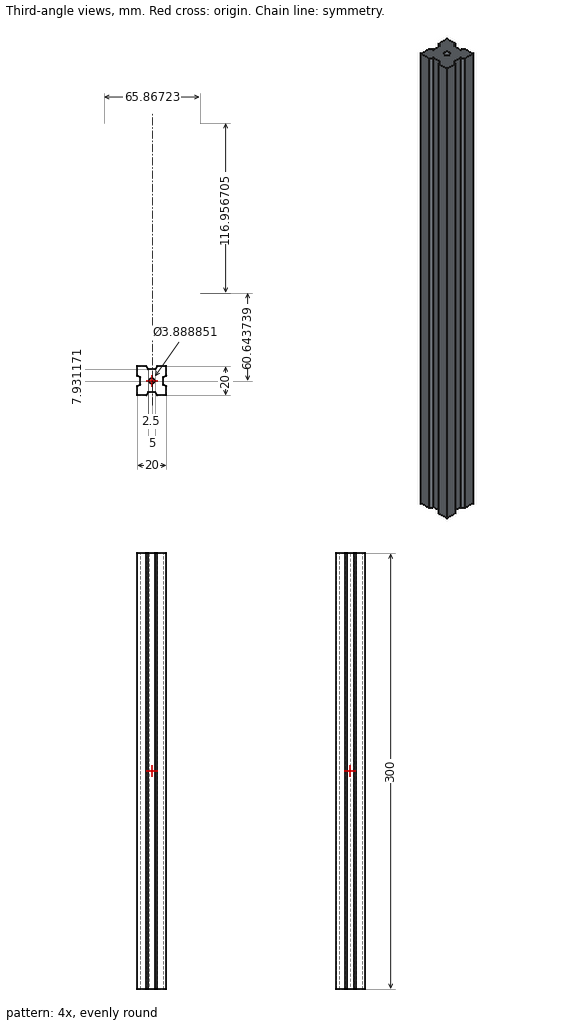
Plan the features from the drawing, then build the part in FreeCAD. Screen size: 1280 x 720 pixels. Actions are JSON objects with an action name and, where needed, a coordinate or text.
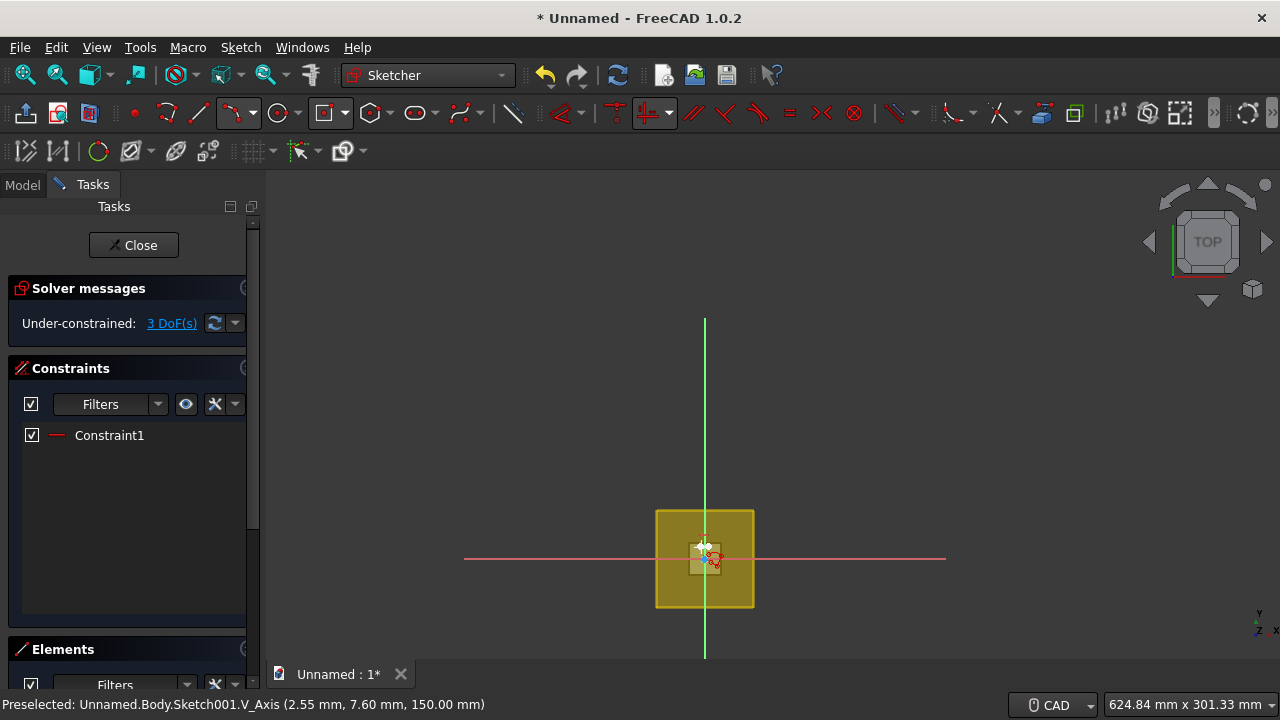
{"action": "left_click", "coordinate": [758, 461]}
{"action": "left_click", "coordinate": [758, 271]}
{"action": "left_click", "coordinate": [651, 271]}
{"action": "left_click", "coordinate": [651, 461]}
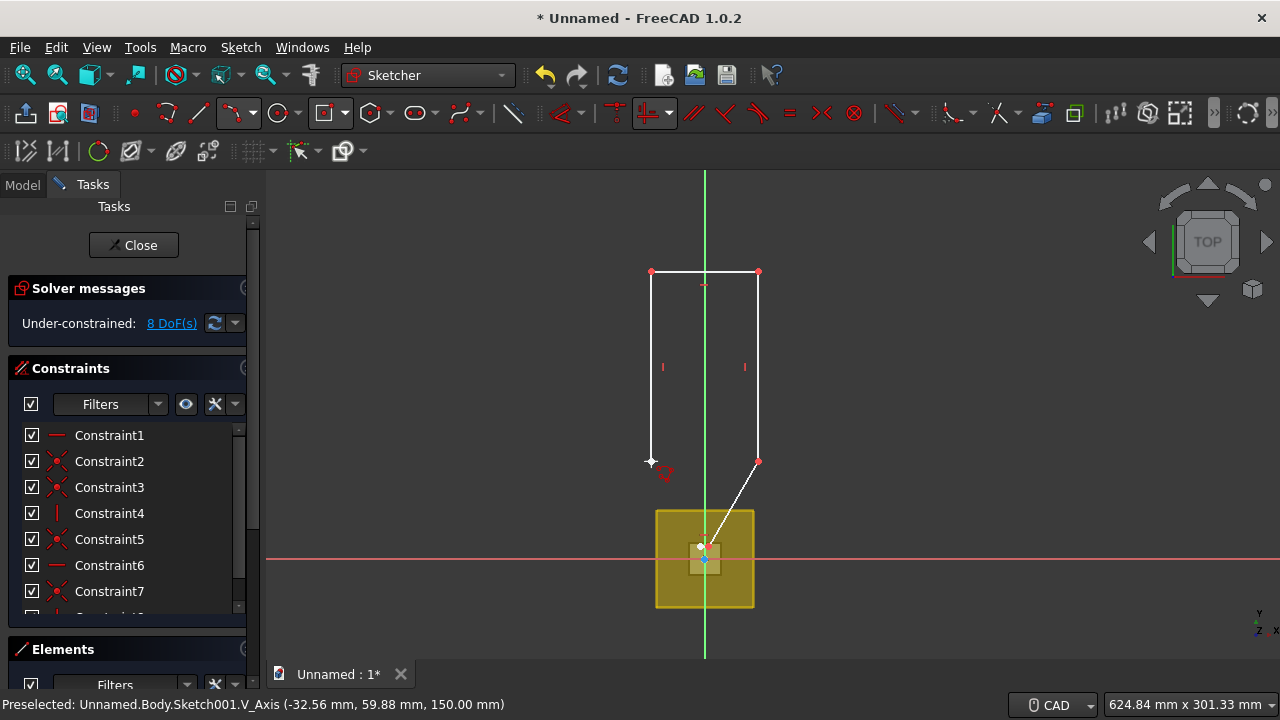
{"action": "scroll", "coordinate": [701, 546], "scroll_direction": "up", "scroll_amount": 7}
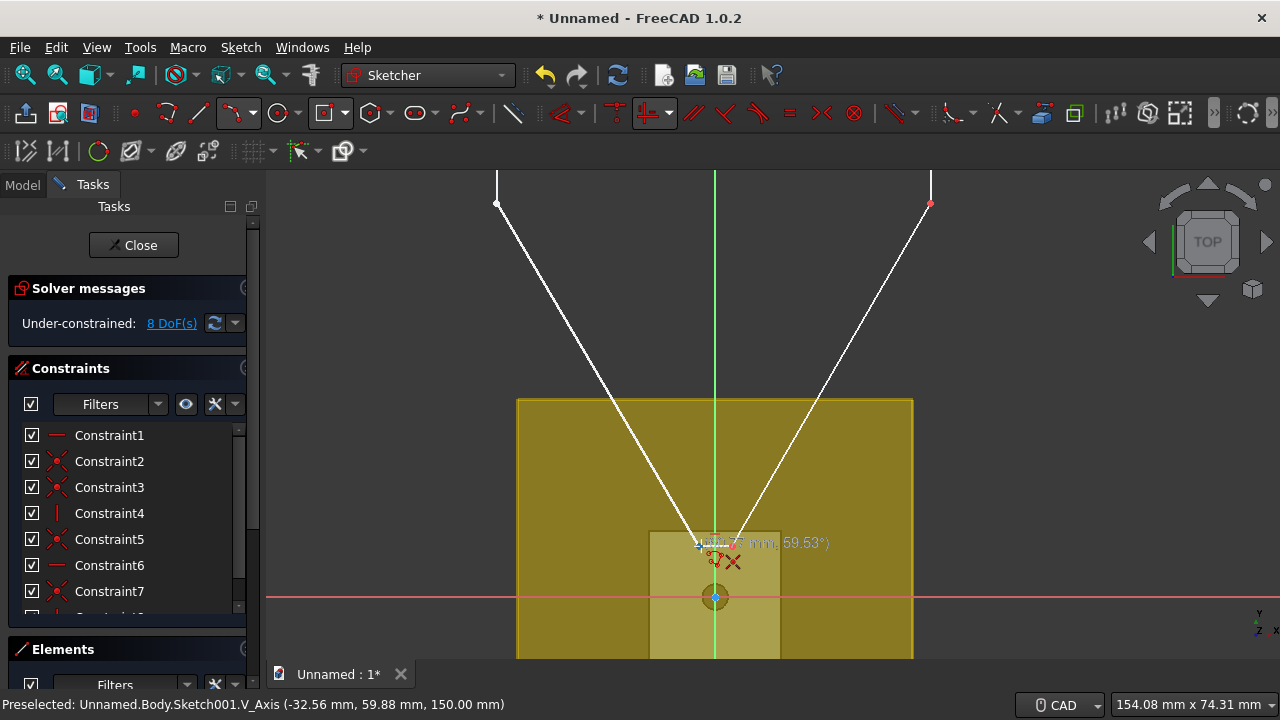
{"action": "left_click", "coordinate": [699, 546]}
{"action": "key", "text": "Escape"}
{"action": "key", "text": "Escape"}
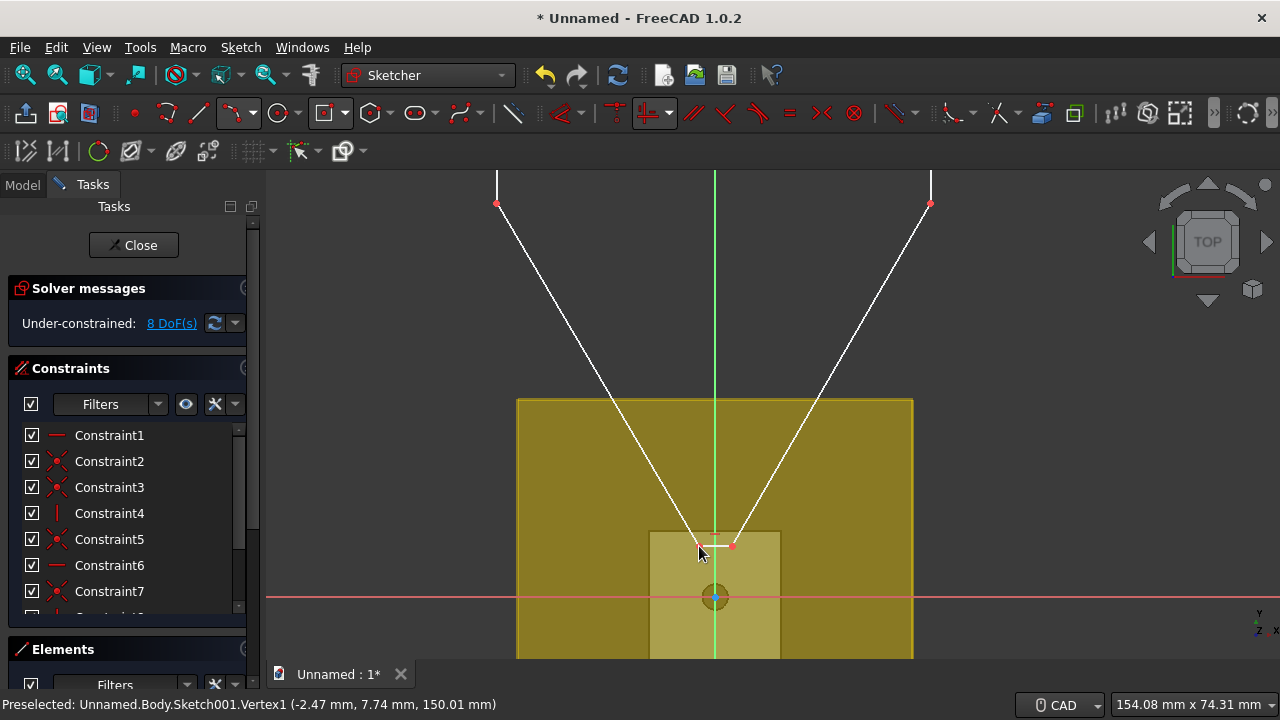
{"action": "scroll", "coordinate": [701, 546], "scroll_direction": "down", "scroll_amount": 7}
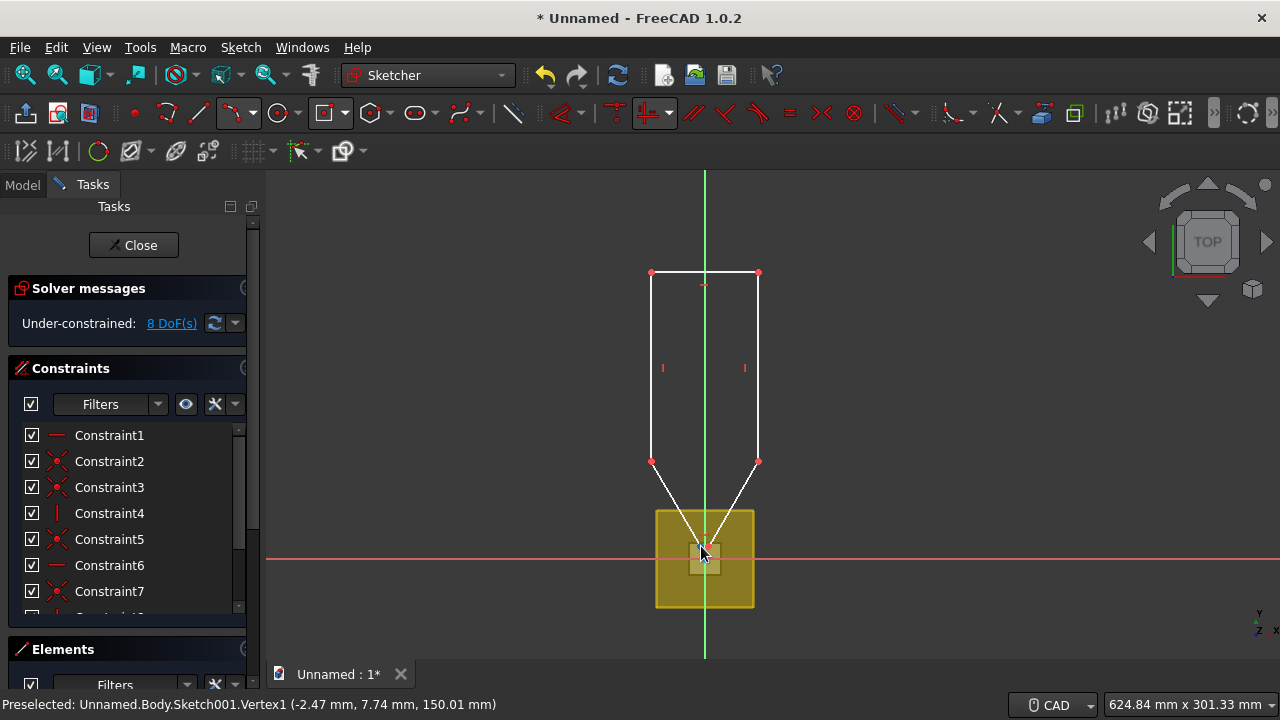
{"action": "left_click", "coordinate": [758, 462]}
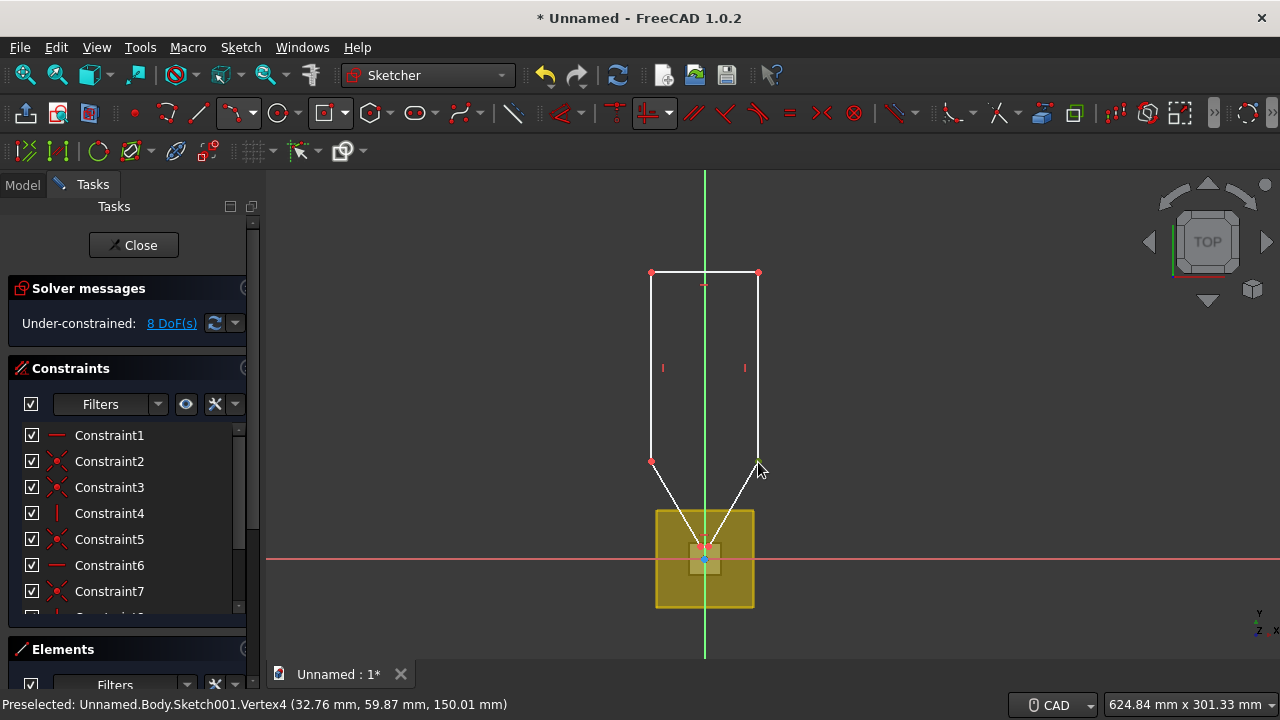
{"action": "left_click", "coordinate": [651, 462]}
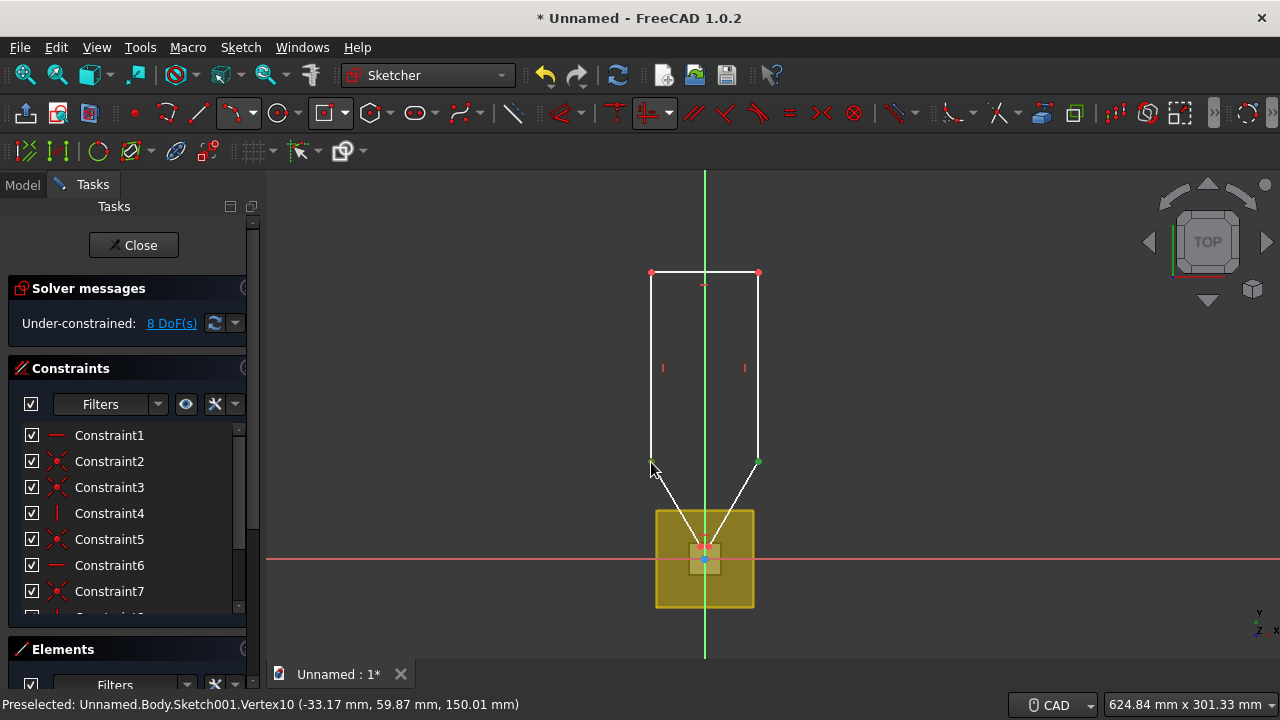
{"action": "left_click", "coordinate": [705, 600]}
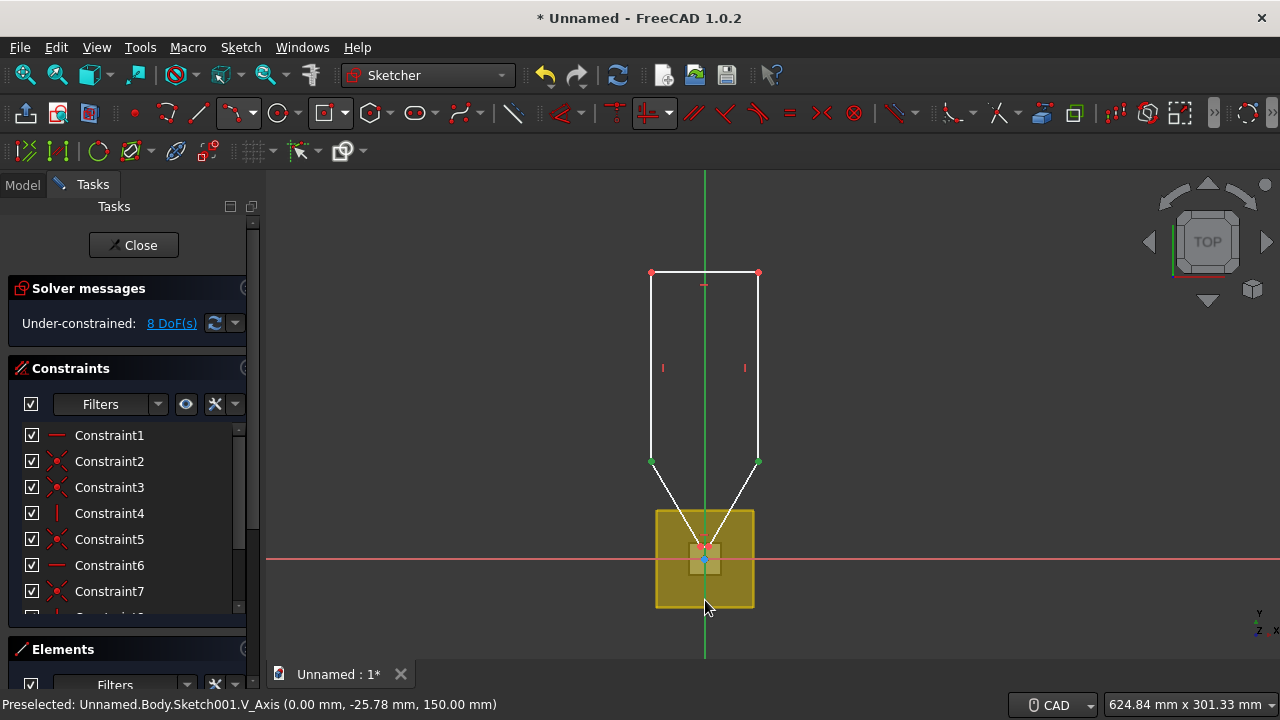
{"action": "left_click", "coordinate": [822, 114]}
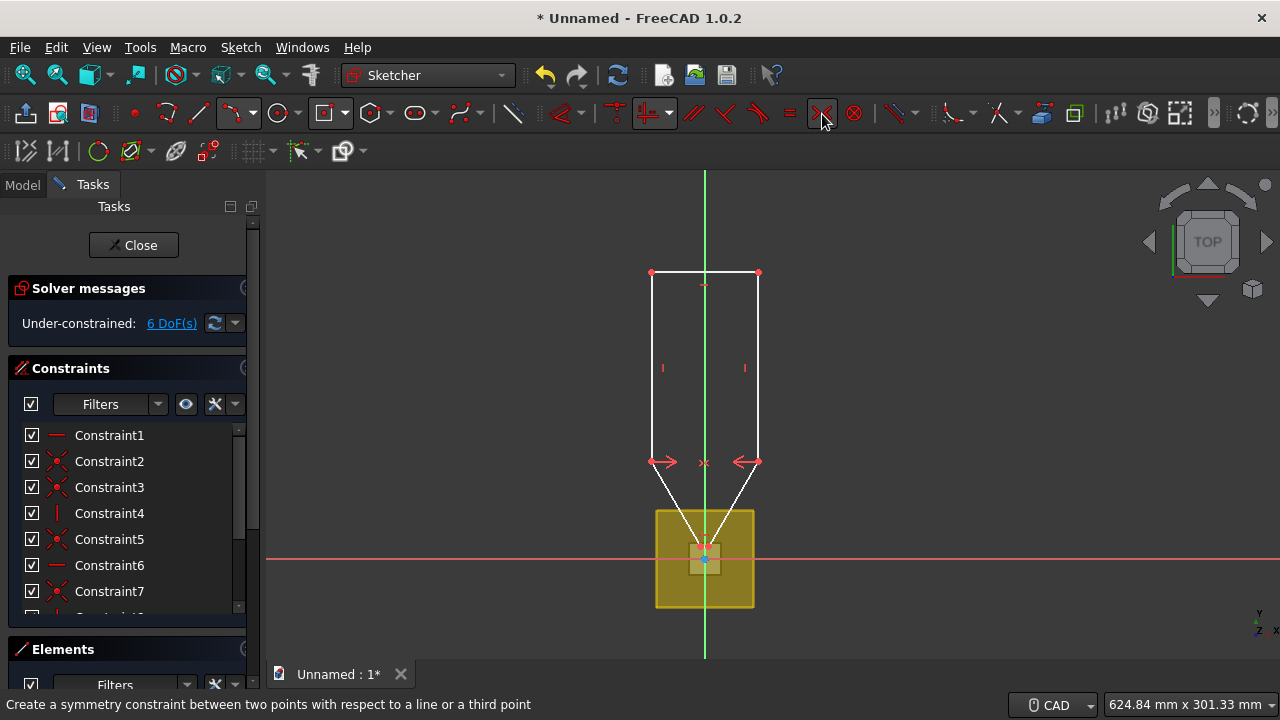
{"action": "left_click", "coordinate": [560, 114]}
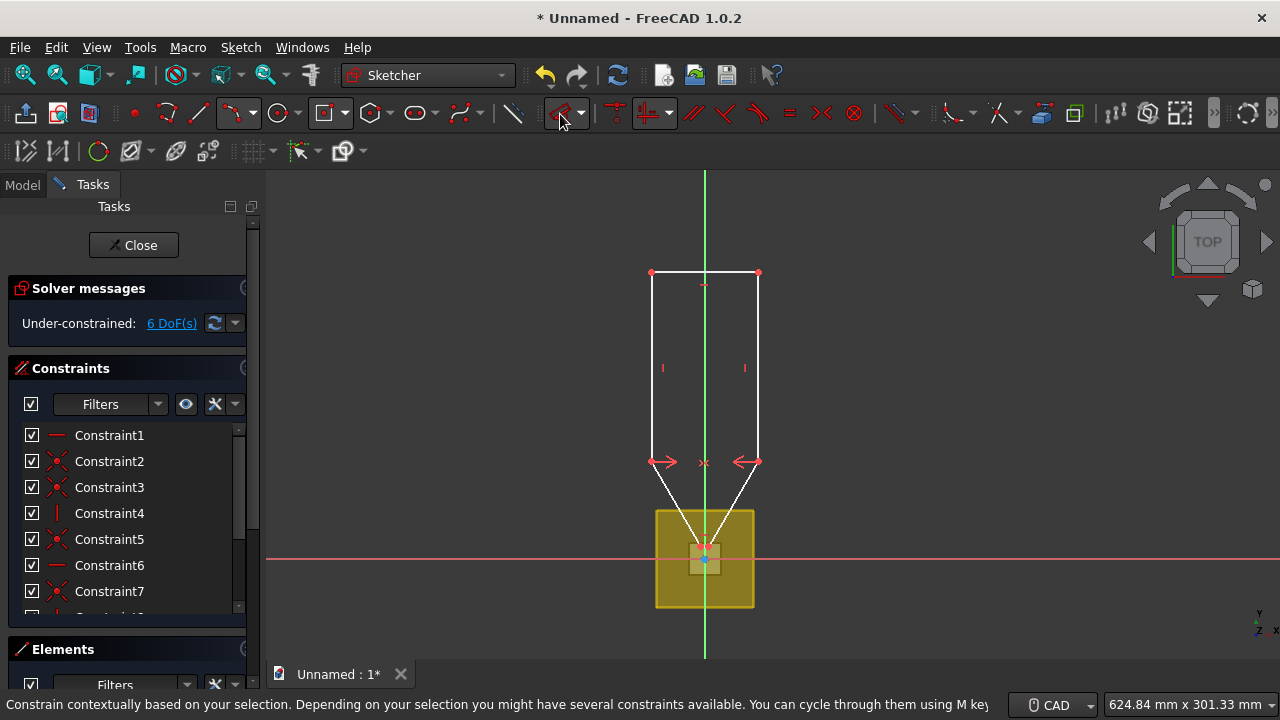
{"action": "scroll", "coordinate": [705, 547], "scroll_direction": "up", "scroll_amount": 8}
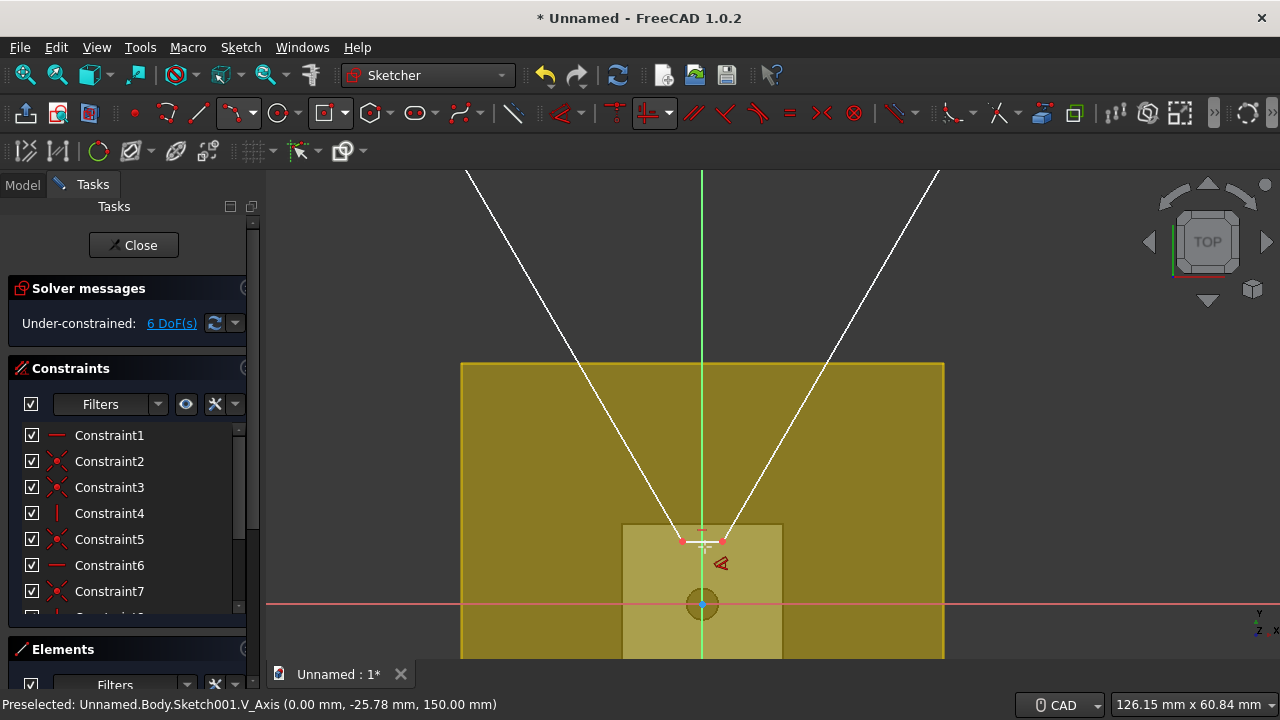
{"action": "left_click", "coordinate": [703, 542]}
{"action": "left_click", "coordinate": [689, 576]}